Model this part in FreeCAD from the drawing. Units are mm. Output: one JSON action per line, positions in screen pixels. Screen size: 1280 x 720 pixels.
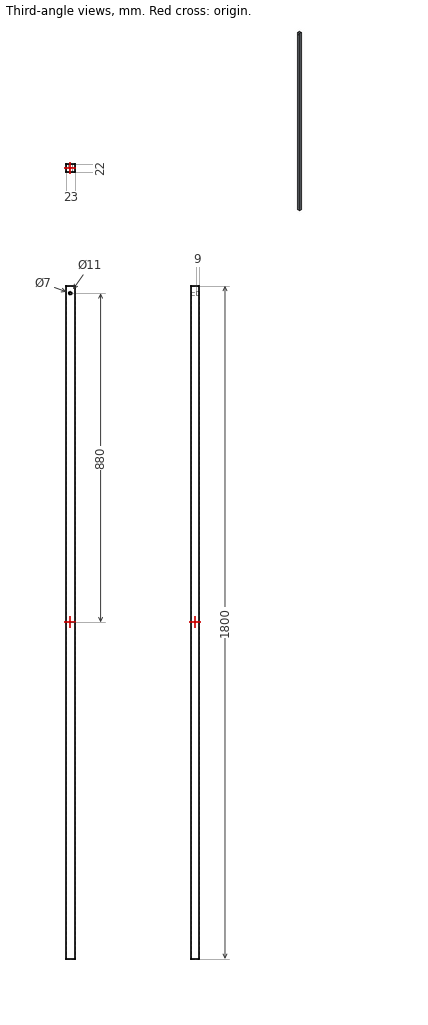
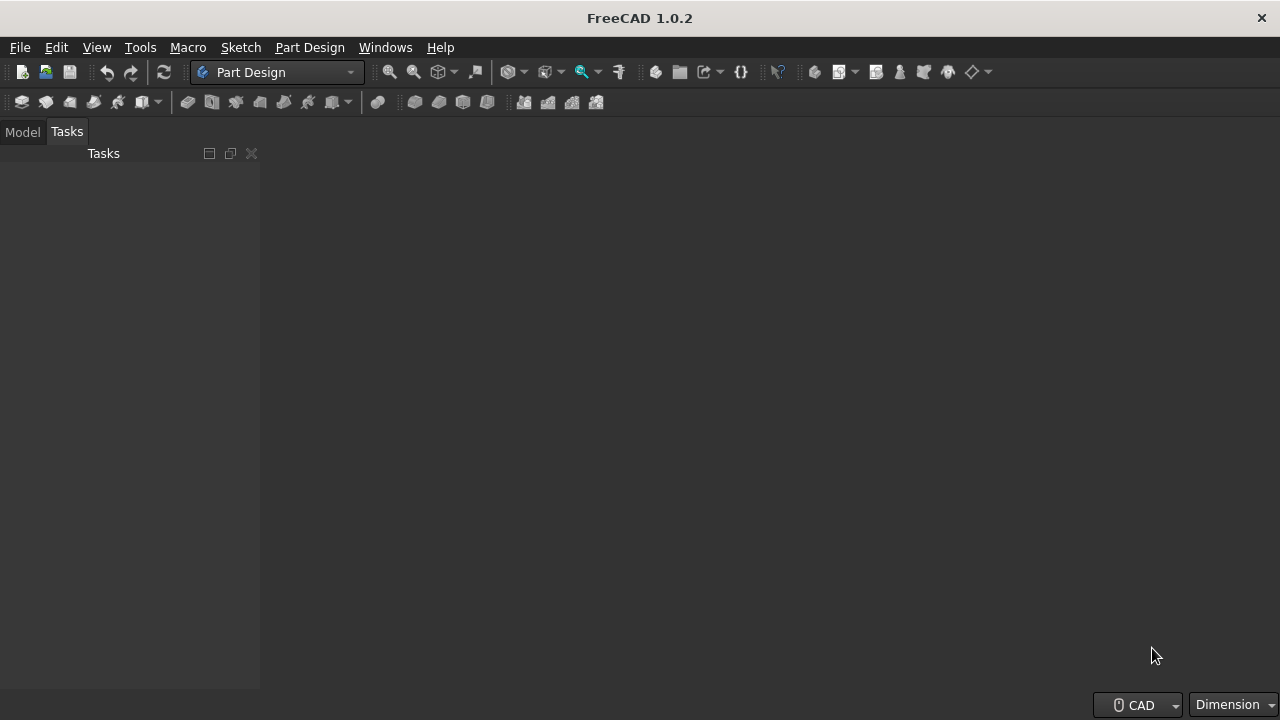
{"action": "left_click", "coordinate": [22, 72]}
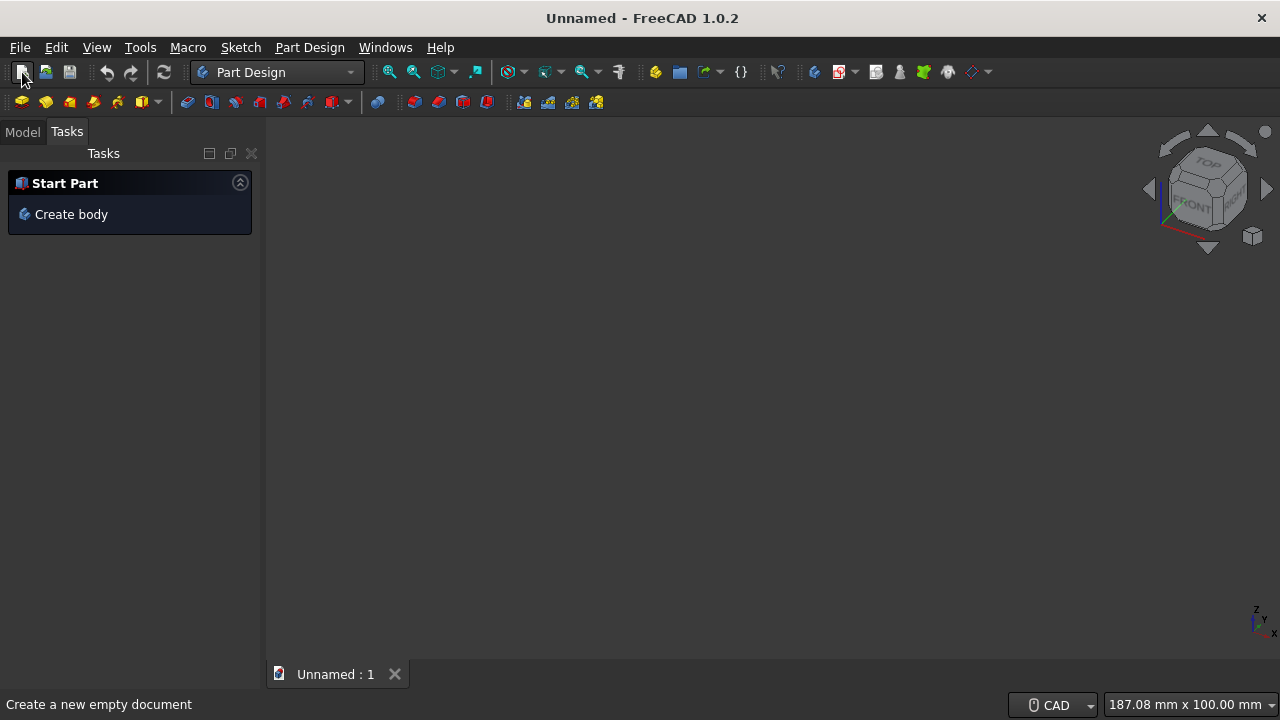
{"action": "left_click", "coordinate": [840, 72]}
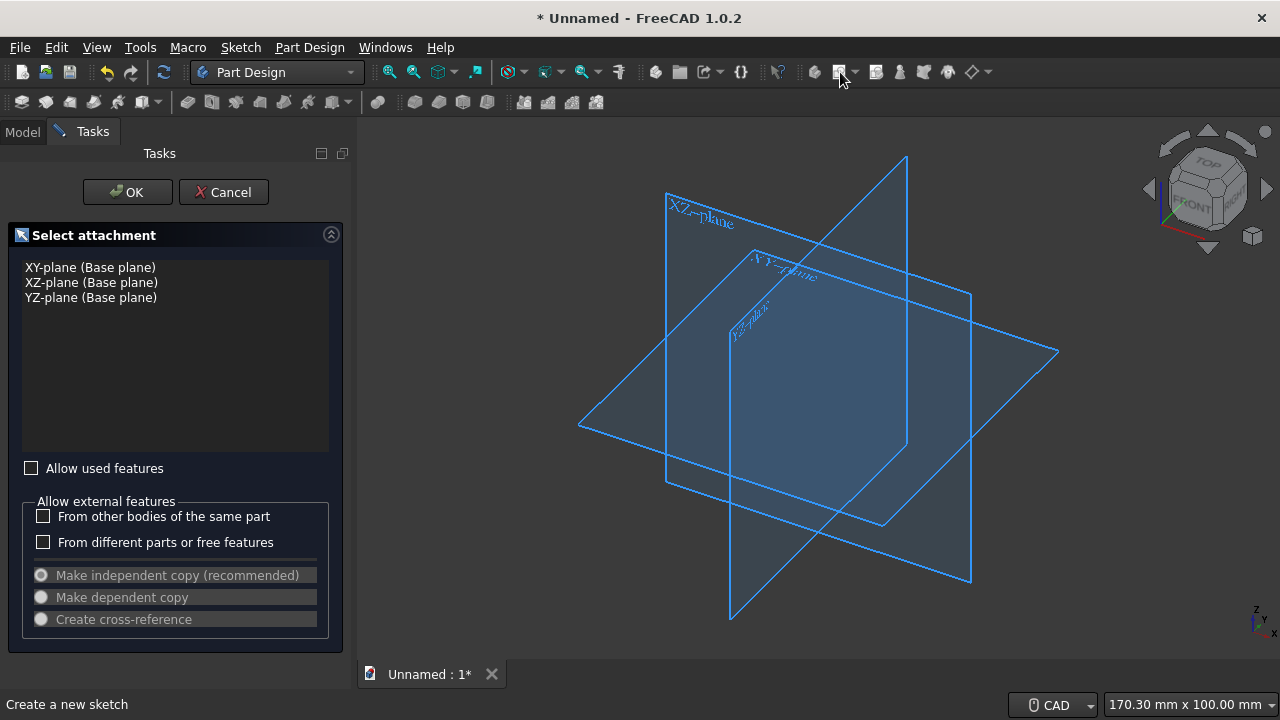
{"action": "left_click", "coordinate": [82, 268]}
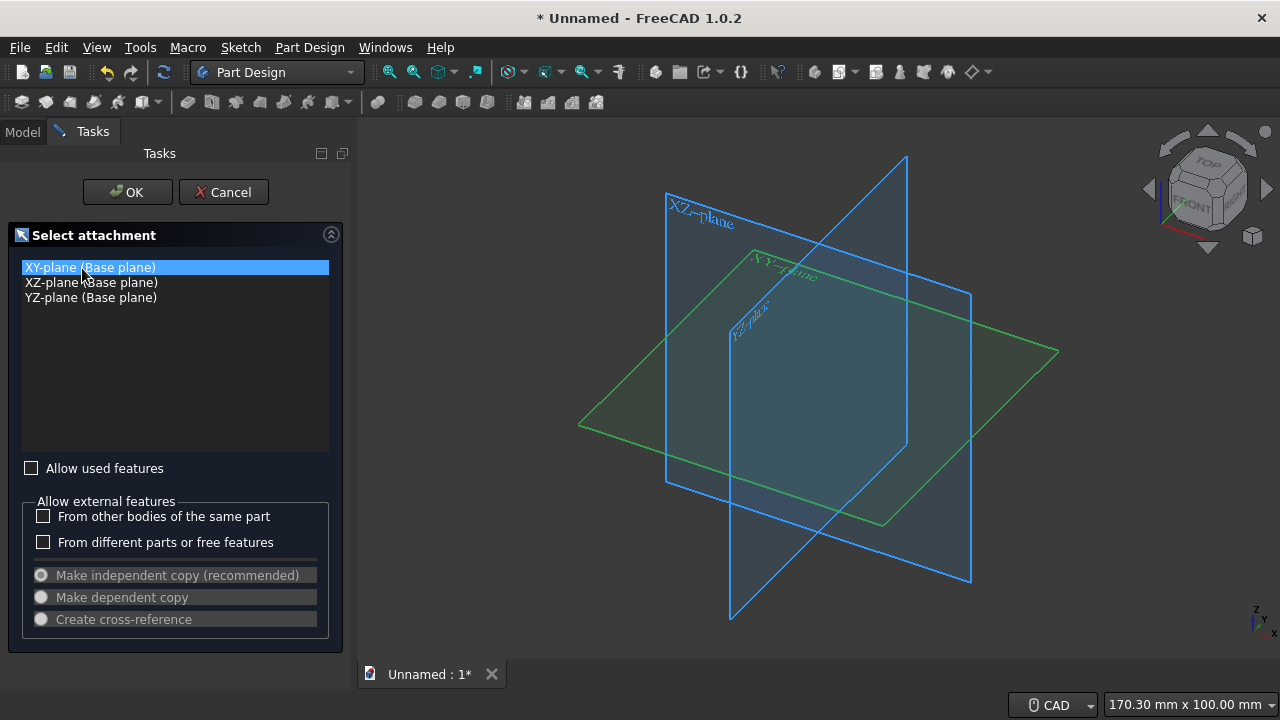
{"action": "left_click", "coordinate": [128, 192]}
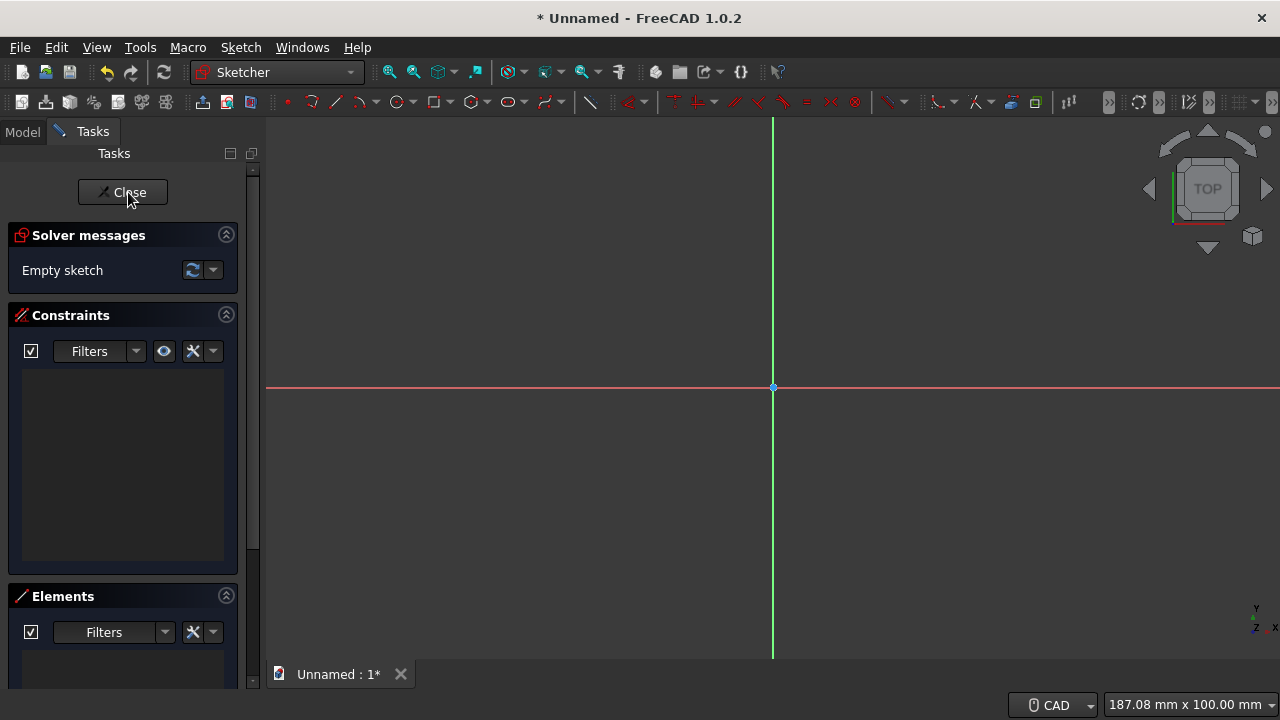
{"action": "scroll", "coordinate": [813, 388], "scroll_direction": "up", "scroll_amount": 5}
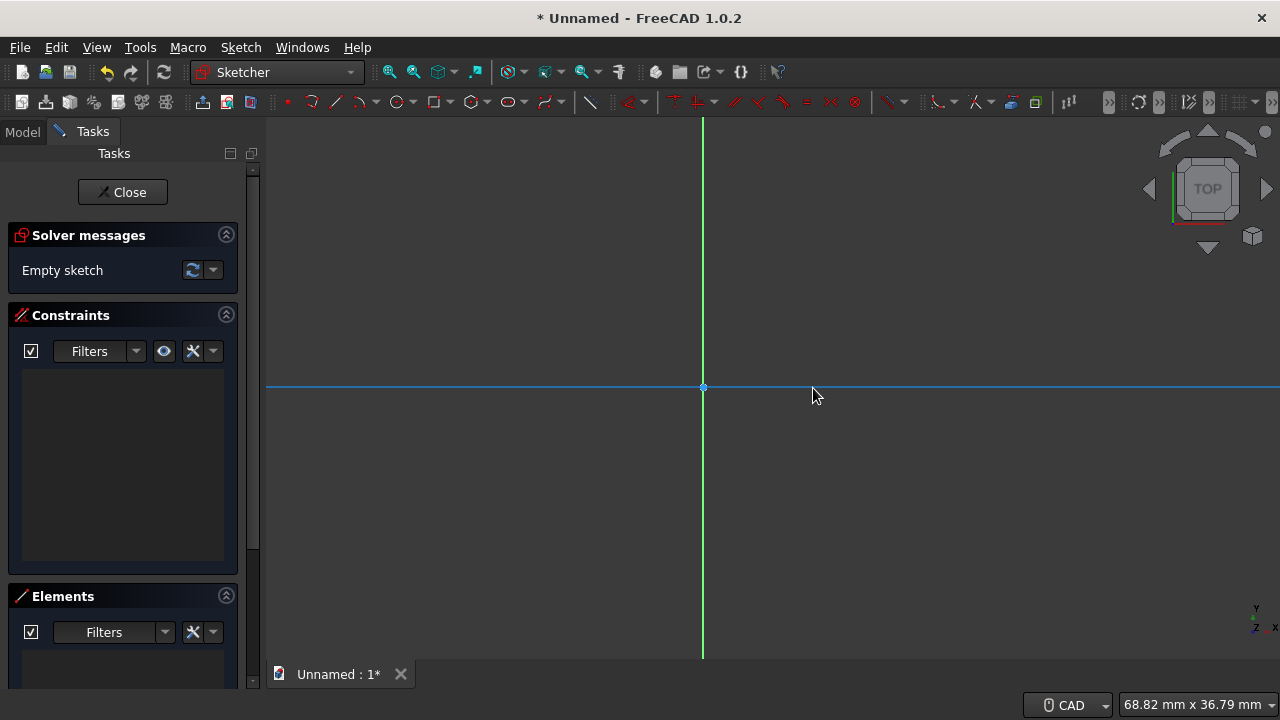
{"action": "left_click", "coordinate": [452, 102]}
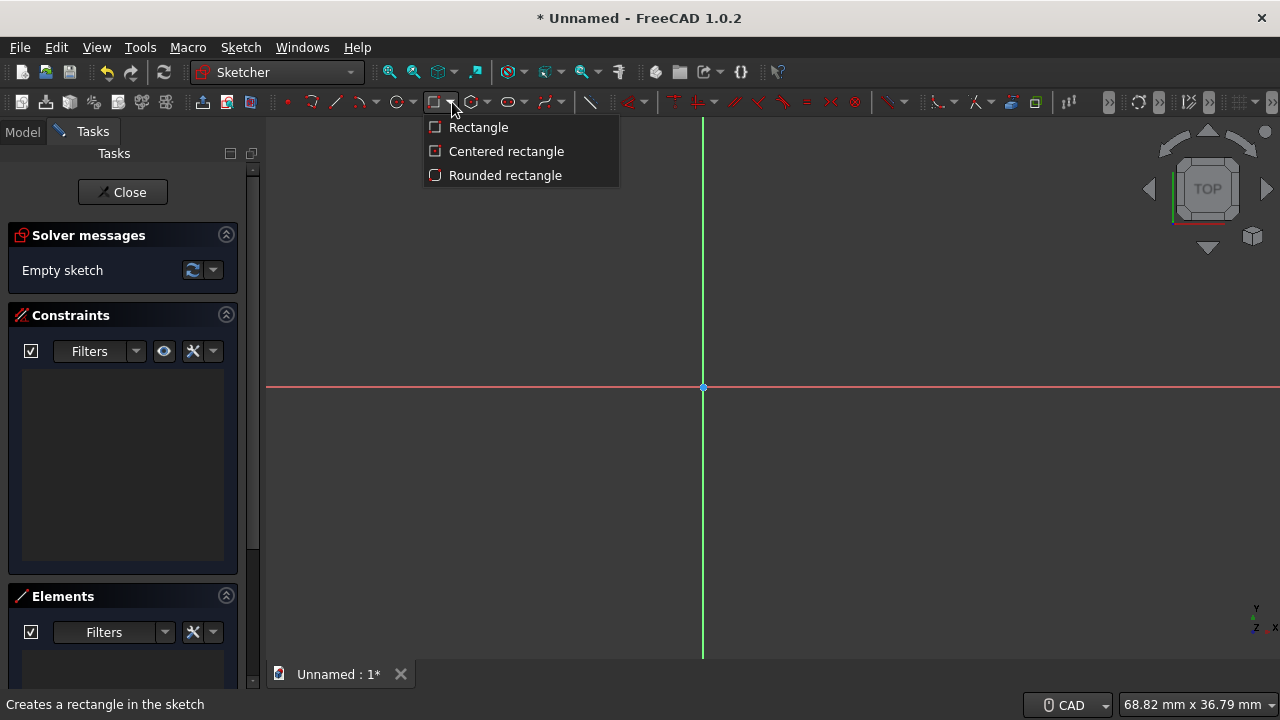
{"action": "left_click", "coordinate": [522, 151]}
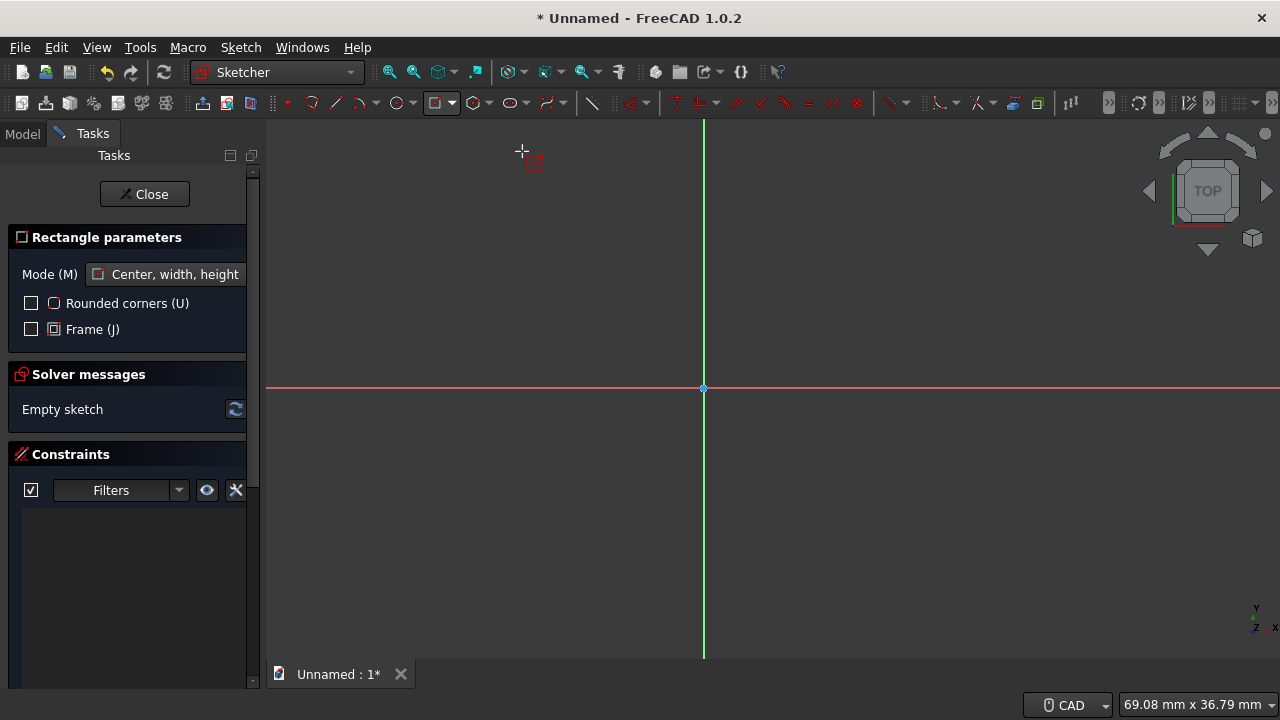
{"action": "left_click", "coordinate": [704, 388]}
{"action": "left_click", "coordinate": [872, 227]}
{"action": "key", "text": "Escape"}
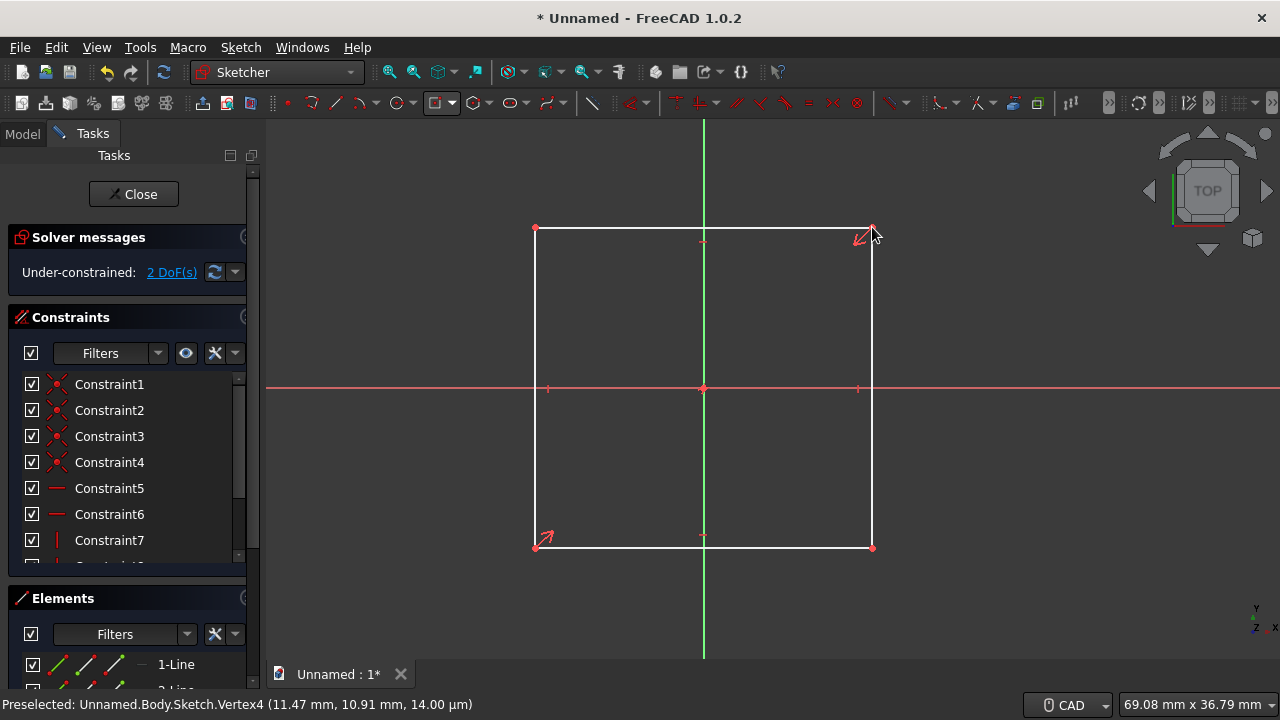
{"action": "left_click", "coordinate": [630, 104]}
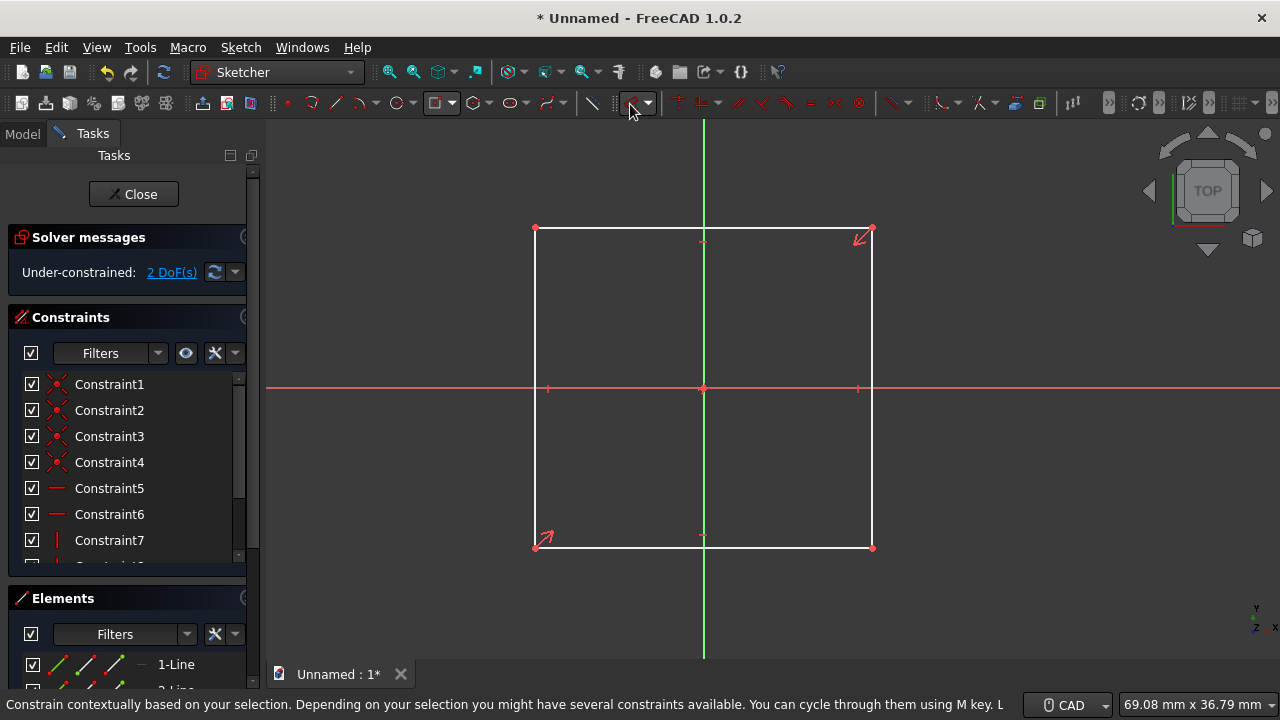
{"action": "left_click", "coordinate": [636, 548]}
{"action": "left_click", "coordinate": [626, 582]}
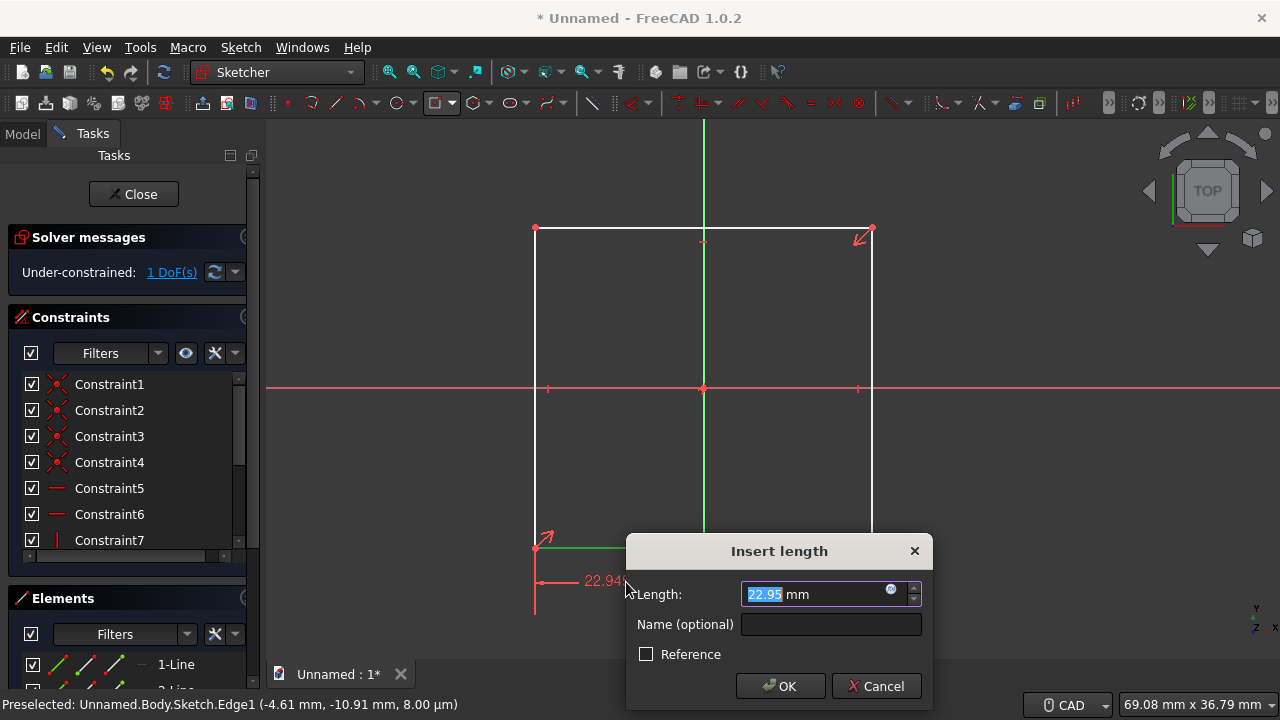
{"action": "type", "text": "23"}
{"action": "key", "text": "Return"}